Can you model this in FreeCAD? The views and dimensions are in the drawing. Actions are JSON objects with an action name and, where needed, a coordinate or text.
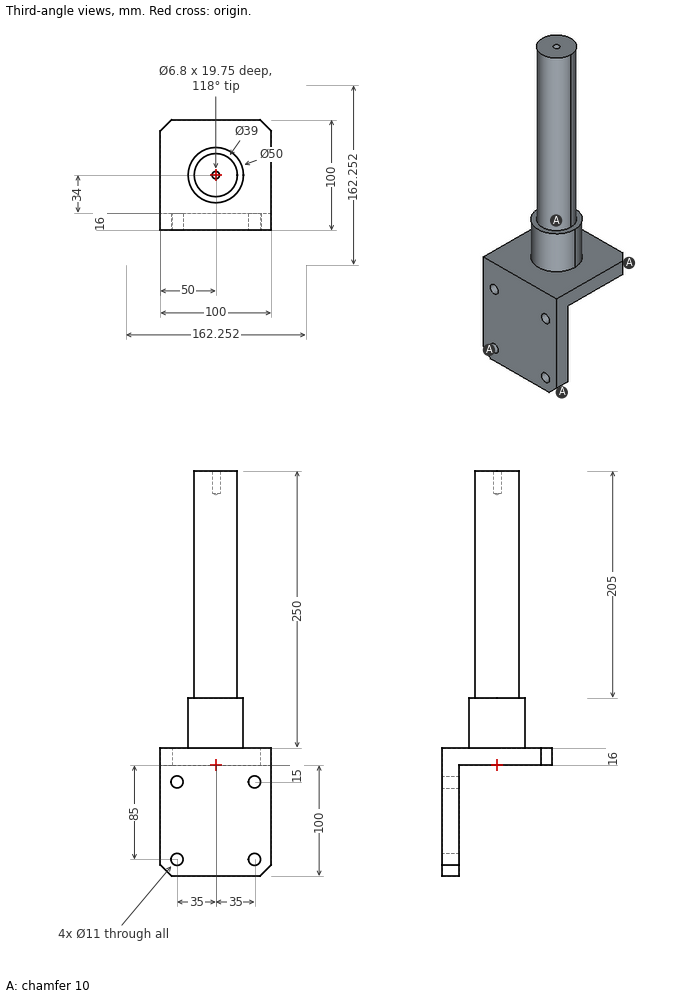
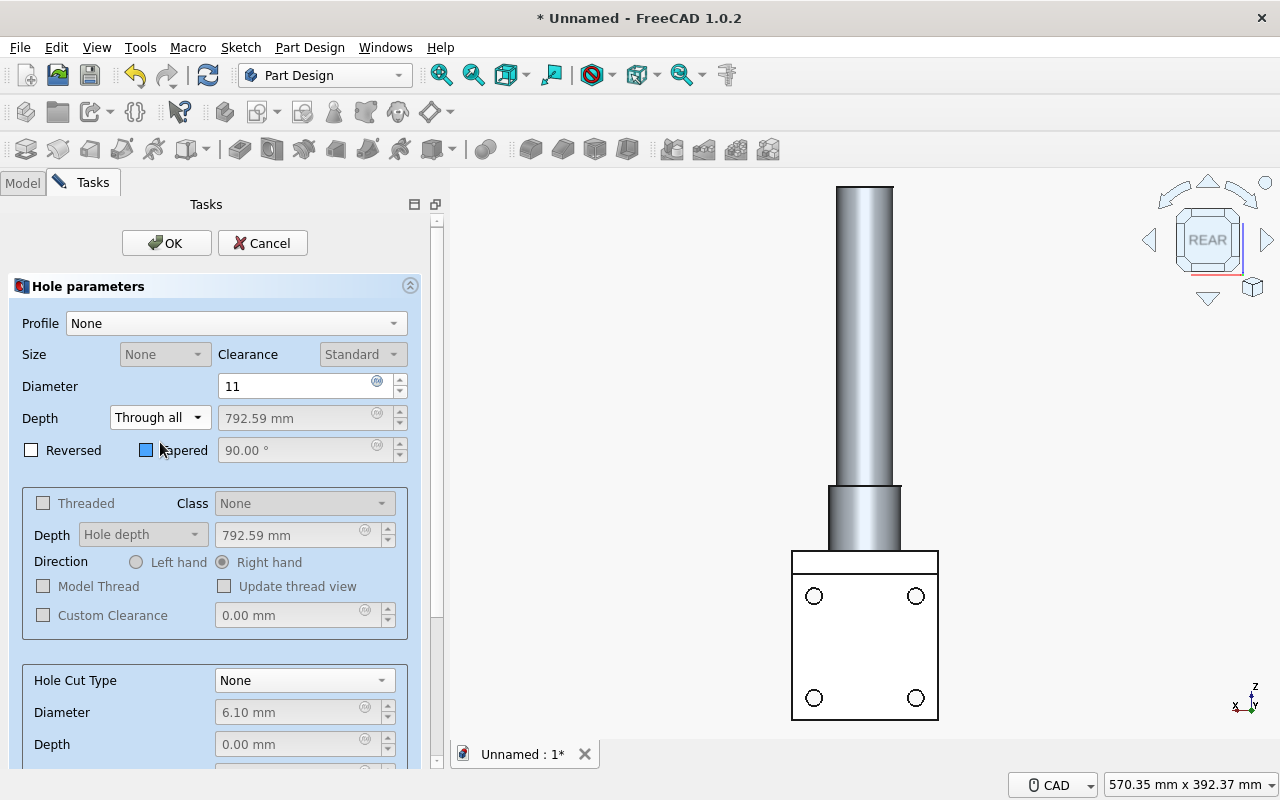
{"action": "left_click", "coordinate": [167, 243]}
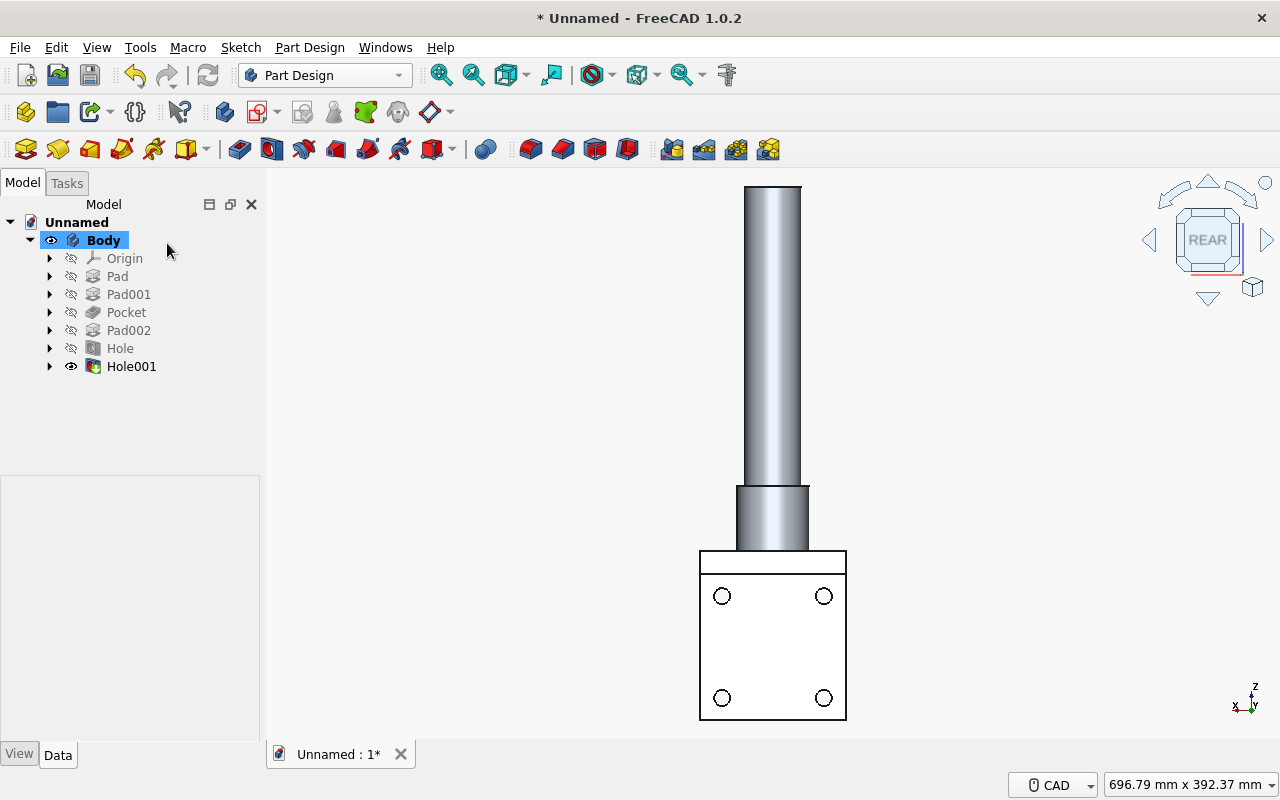
{"action": "left_click", "coordinate": [846, 562]}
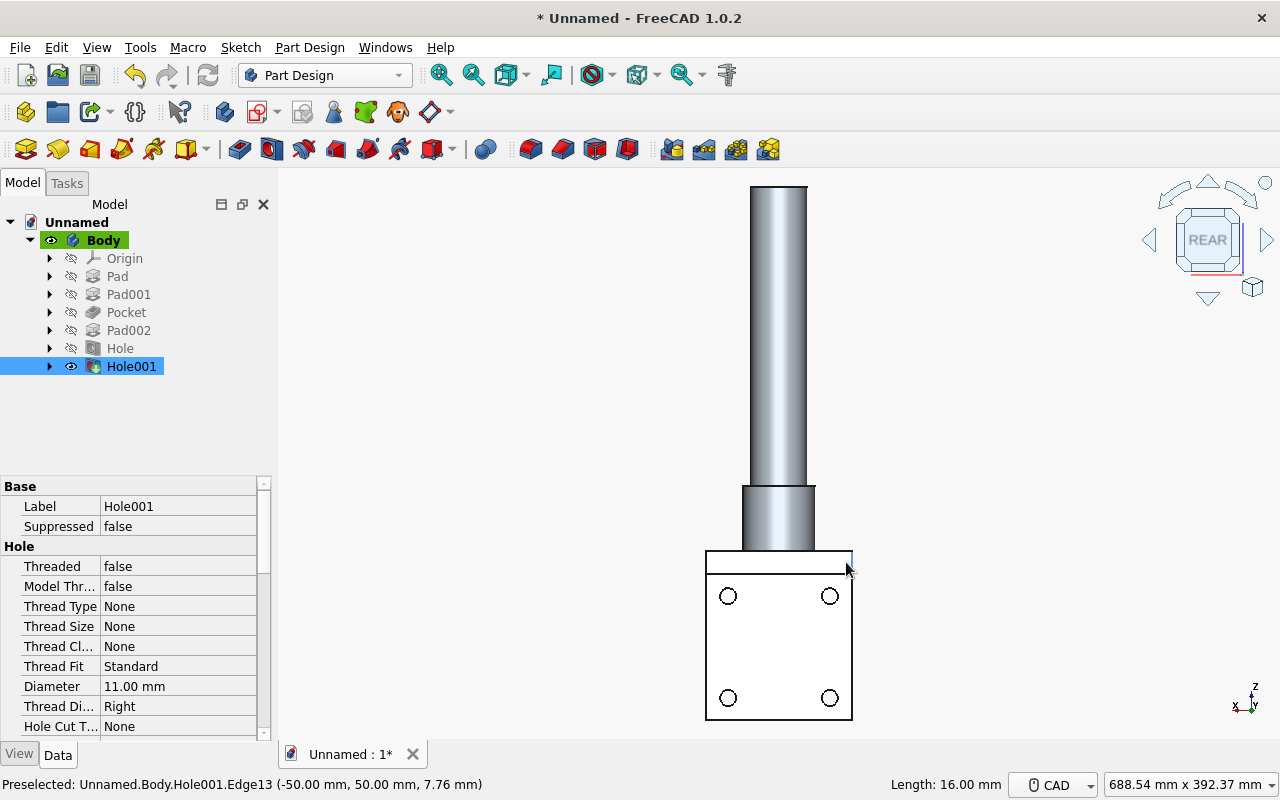
{"action": "key", "text": "0"}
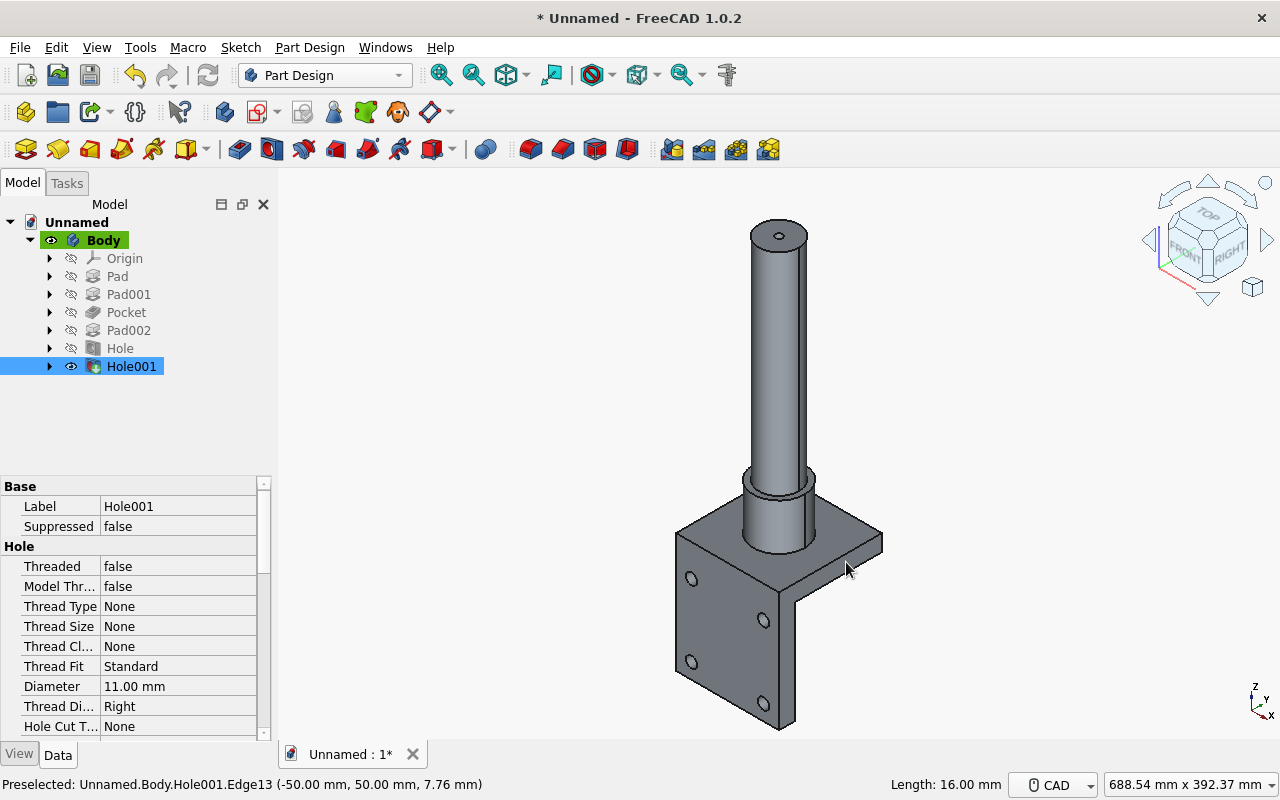
{"action": "key", "text": "2"}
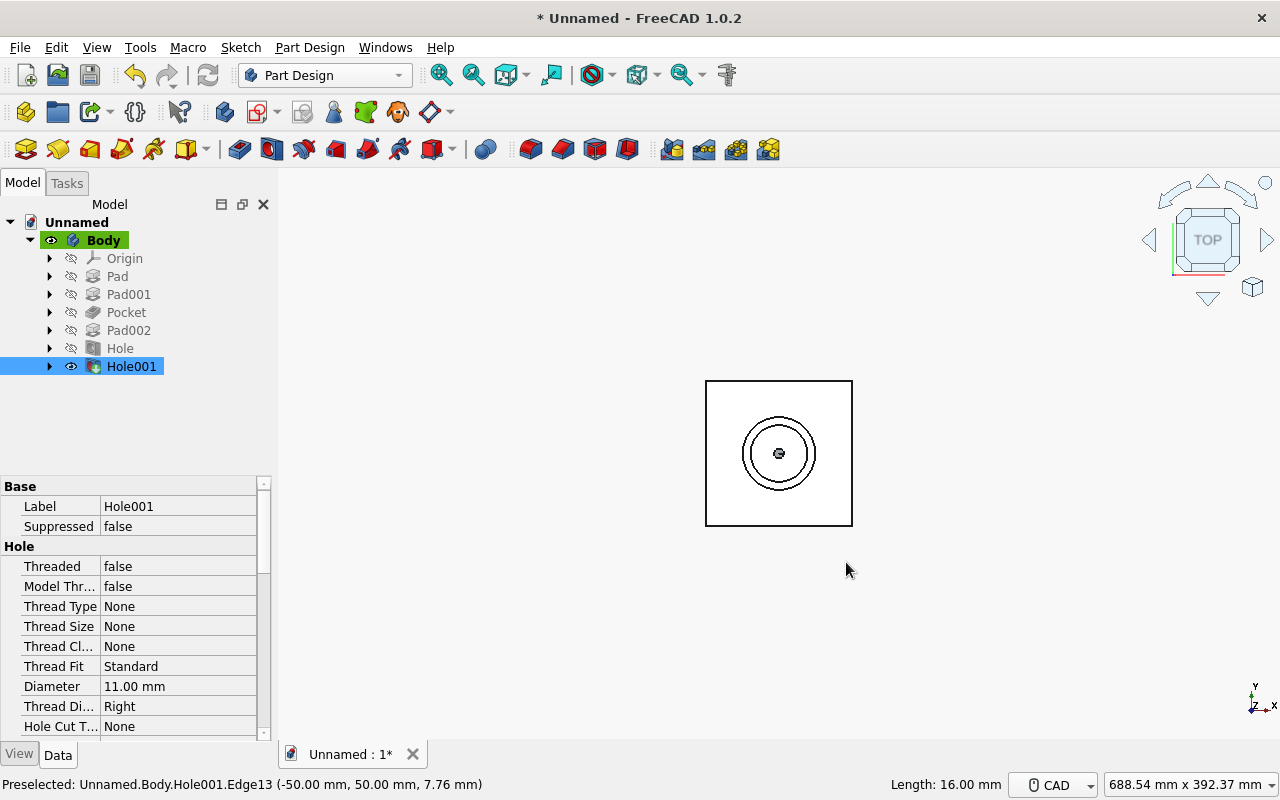
{"action": "left_click", "coordinate": [442, 76]}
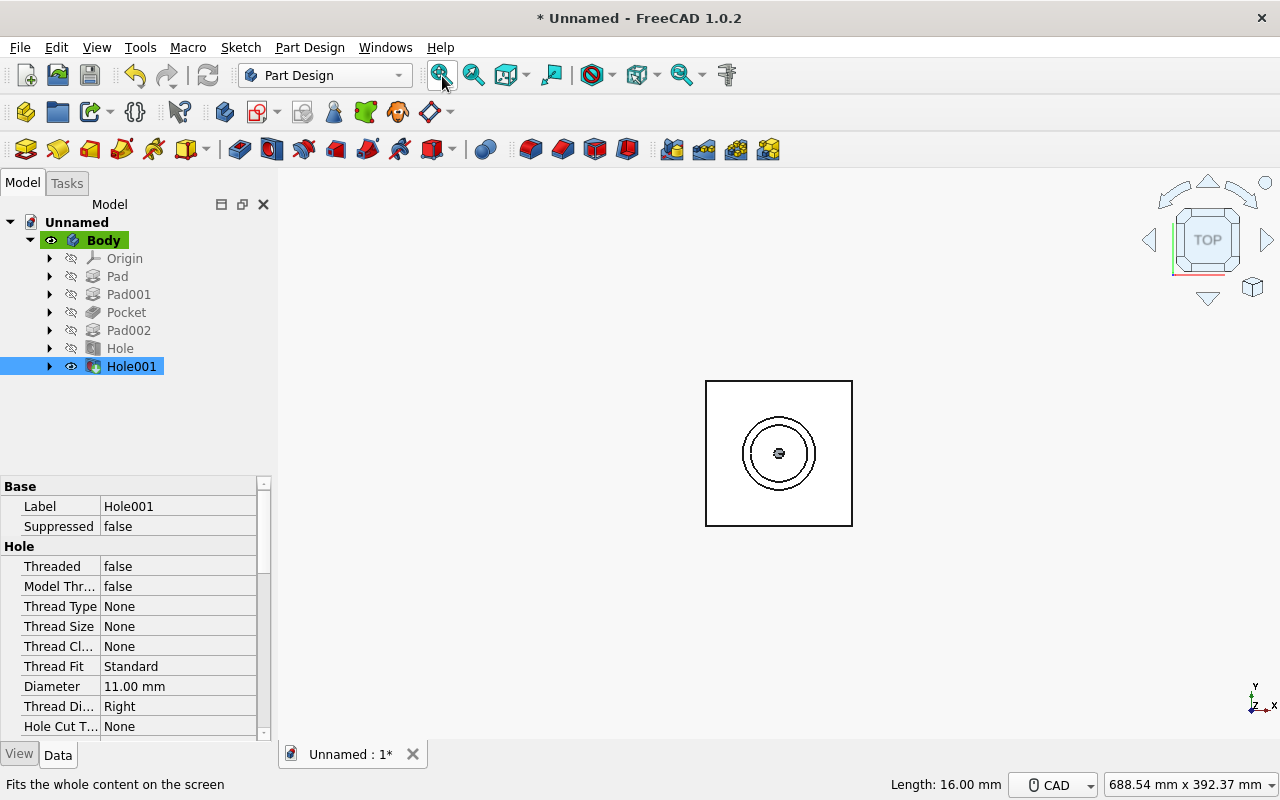
{"action": "key", "text": "1"}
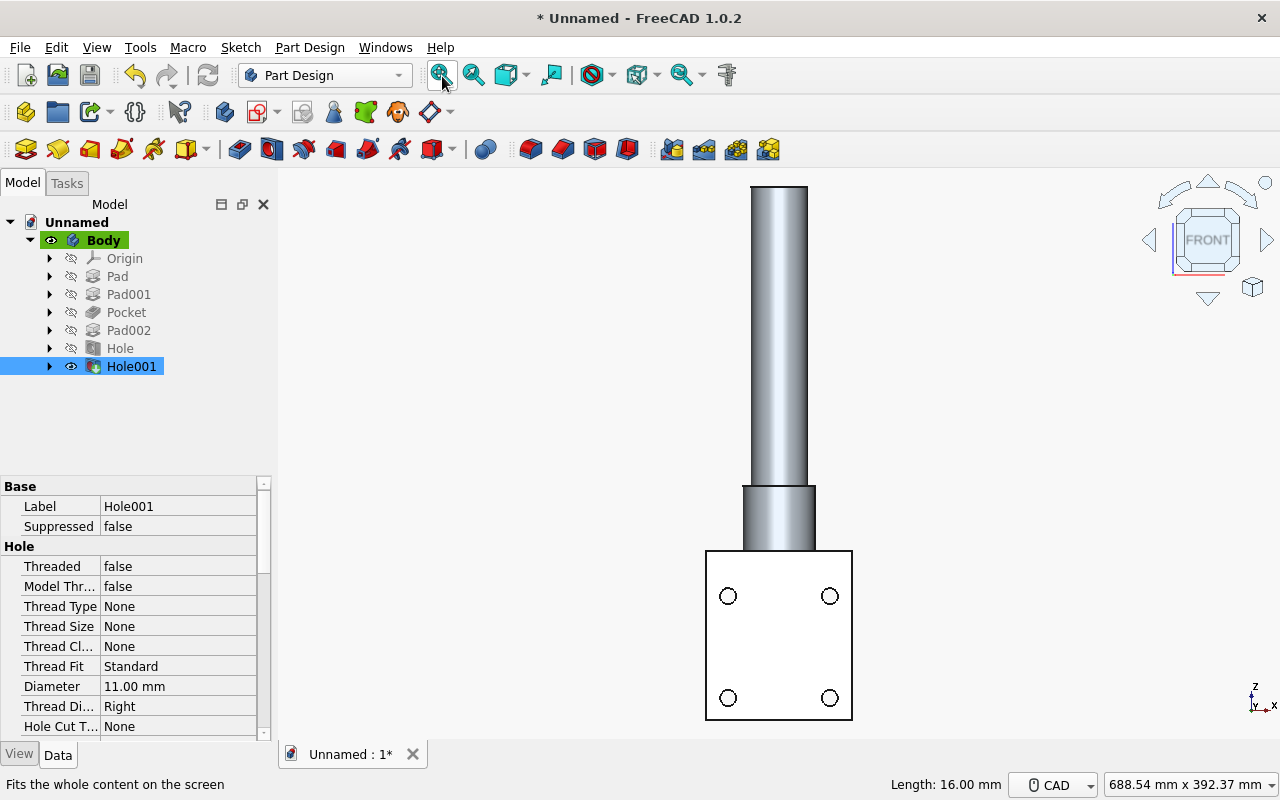
{"action": "key", "text": "3"}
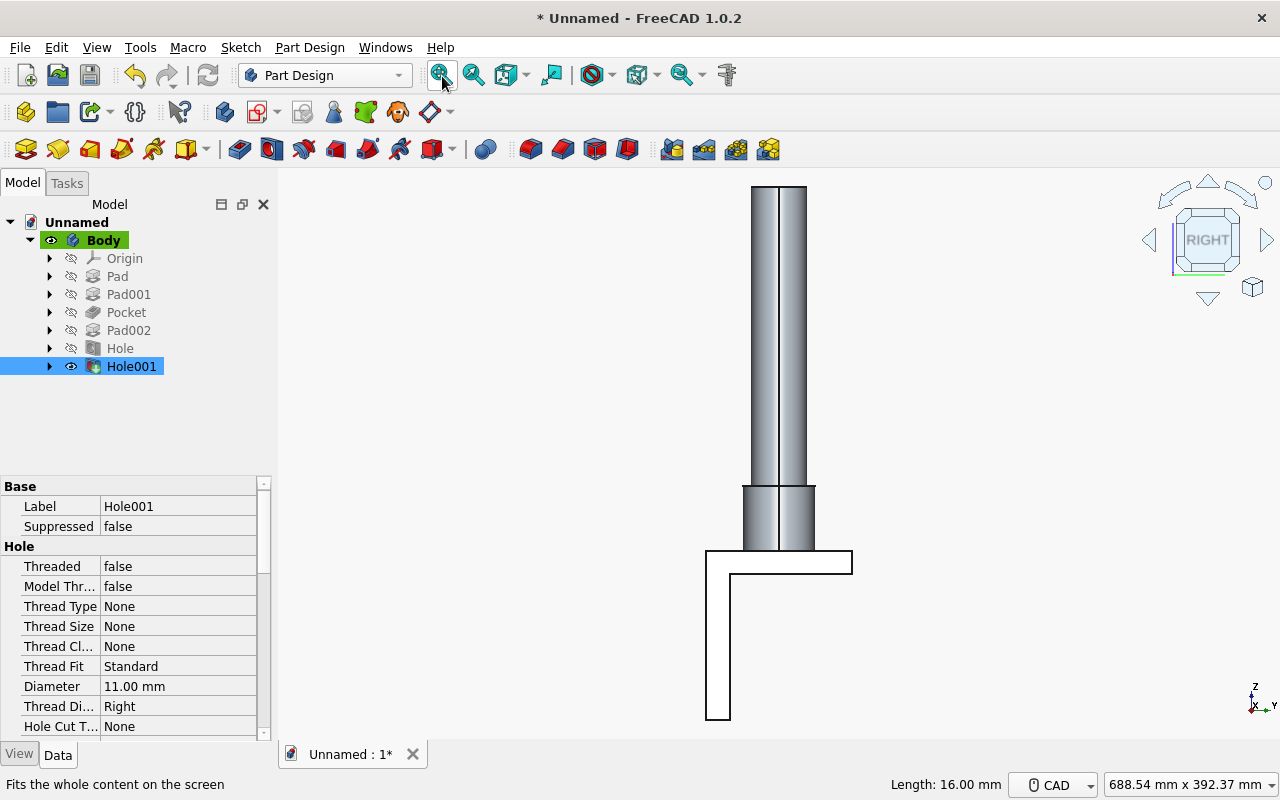
{"action": "left_click", "coordinate": [852, 562], "text": "ctrl"}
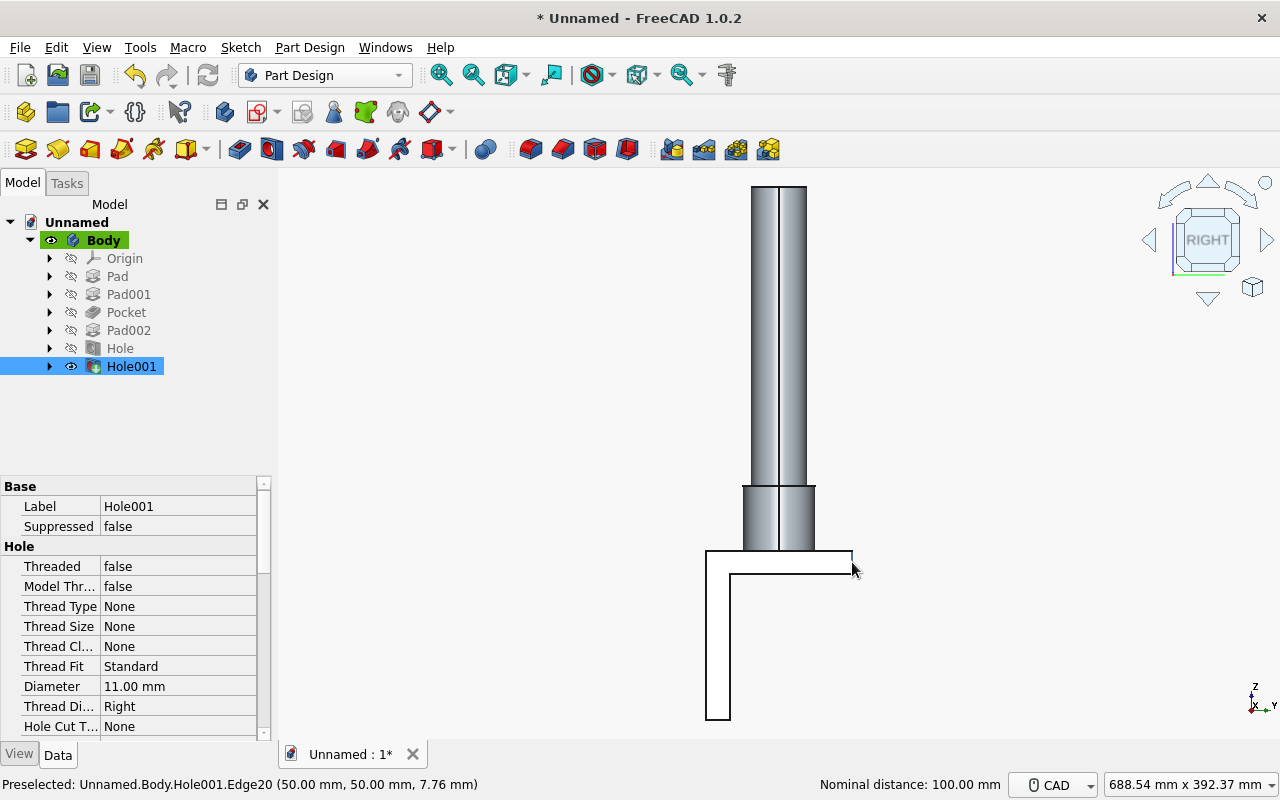
{"action": "key", "text": "5"}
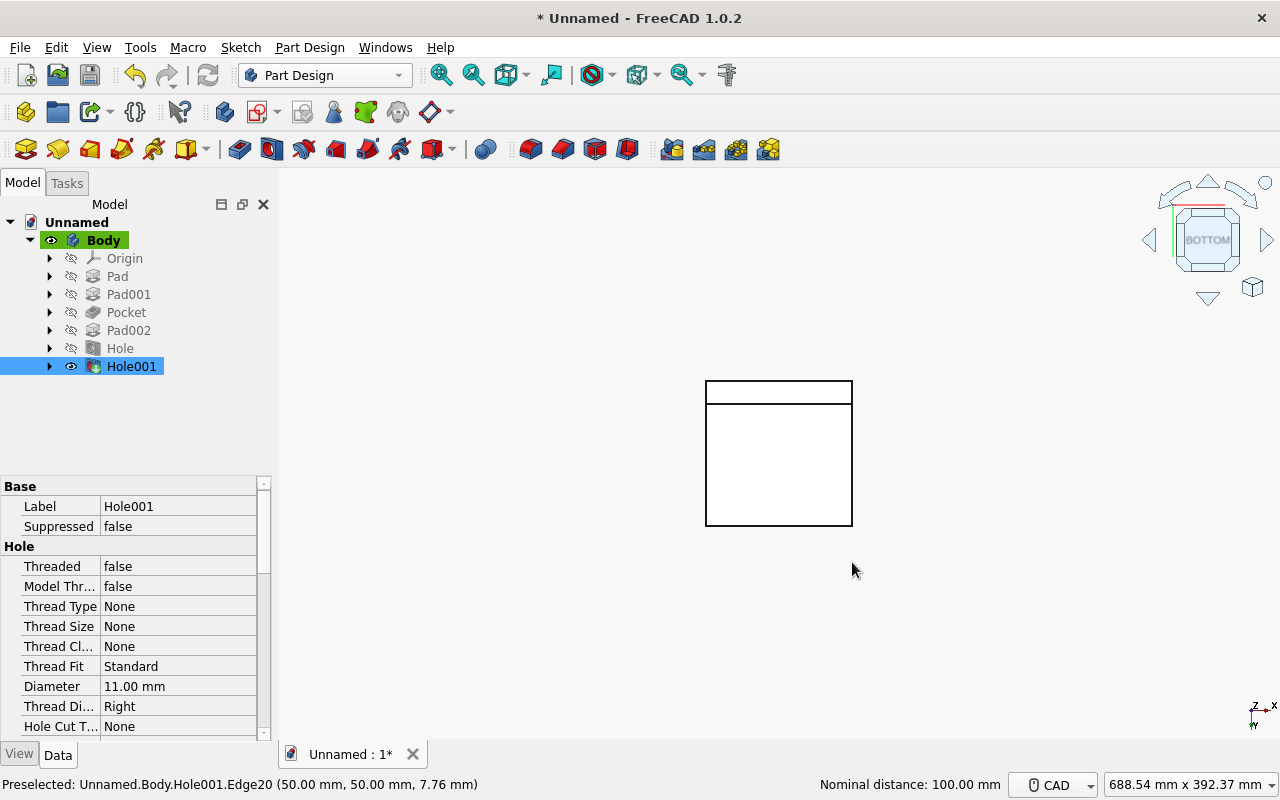
{"action": "key", "text": "v f"}